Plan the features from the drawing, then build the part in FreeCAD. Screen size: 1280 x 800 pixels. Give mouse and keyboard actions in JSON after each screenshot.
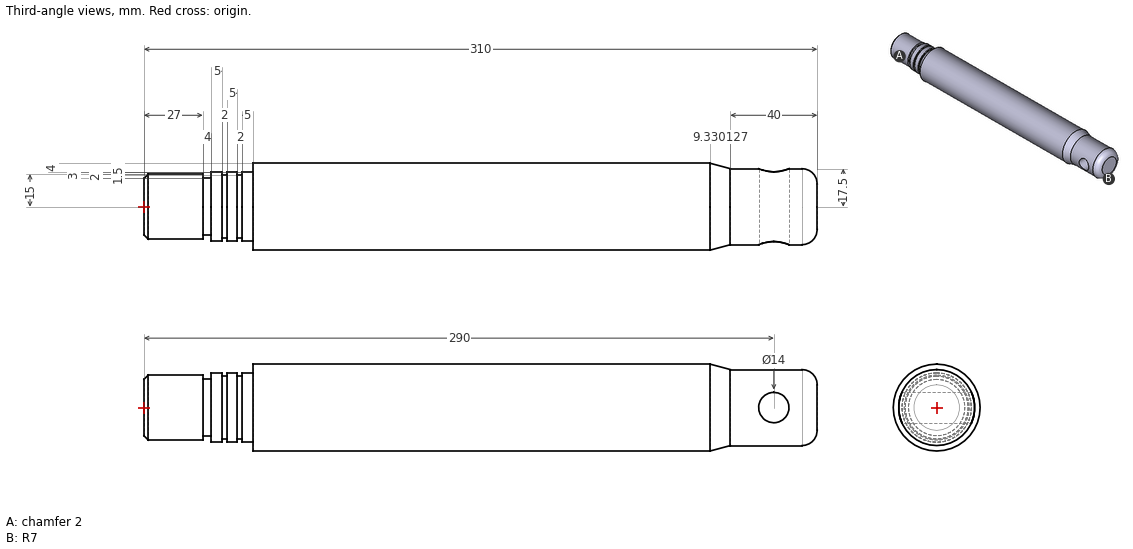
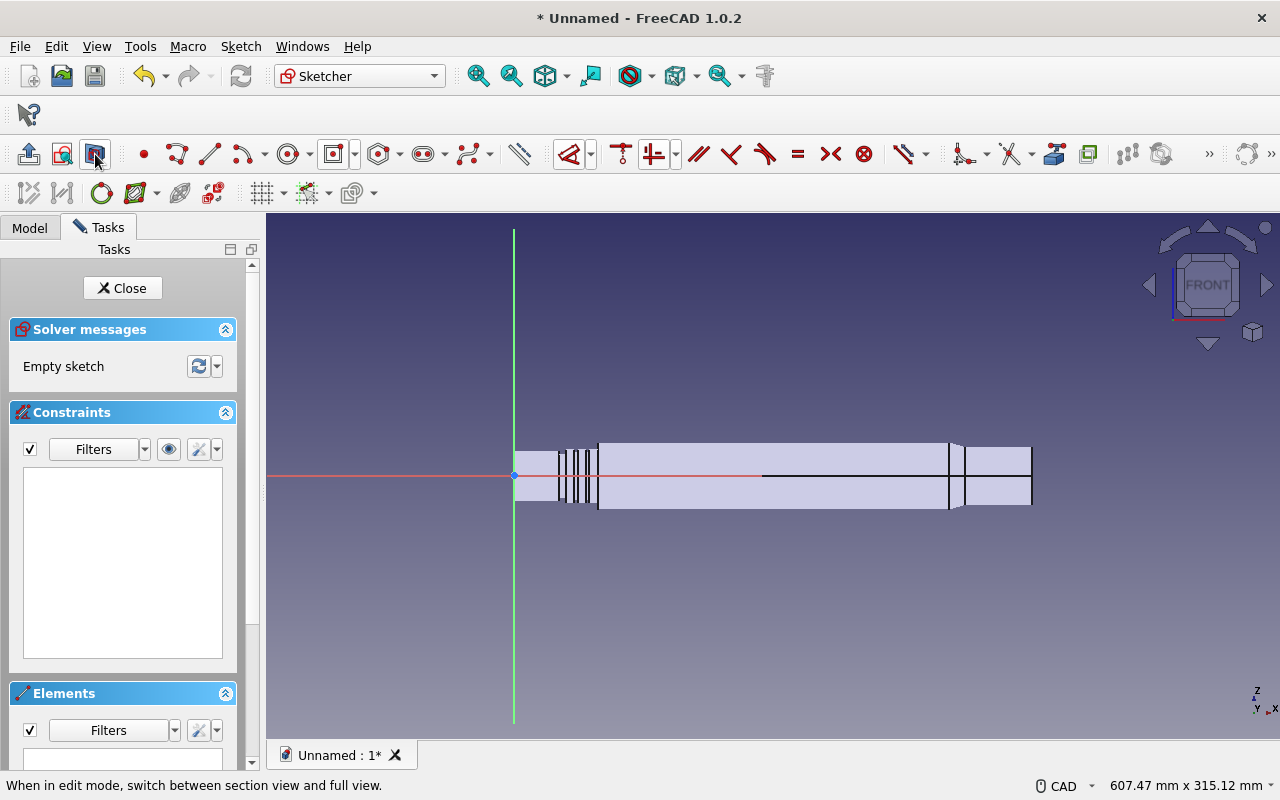
{"action": "scroll", "coordinate": [1022, 476], "scroll_direction": "up", "scroll_amount": 13}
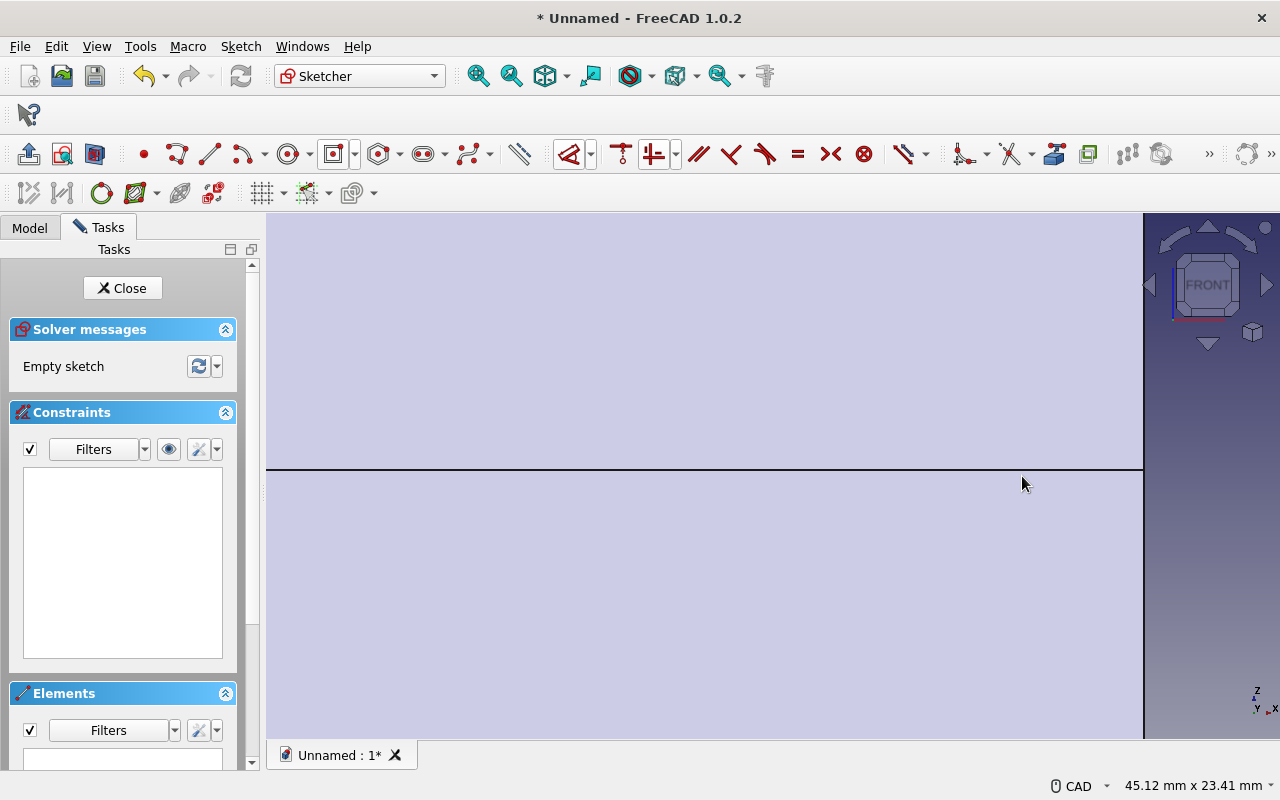
{"action": "left_click", "coordinate": [288, 154]}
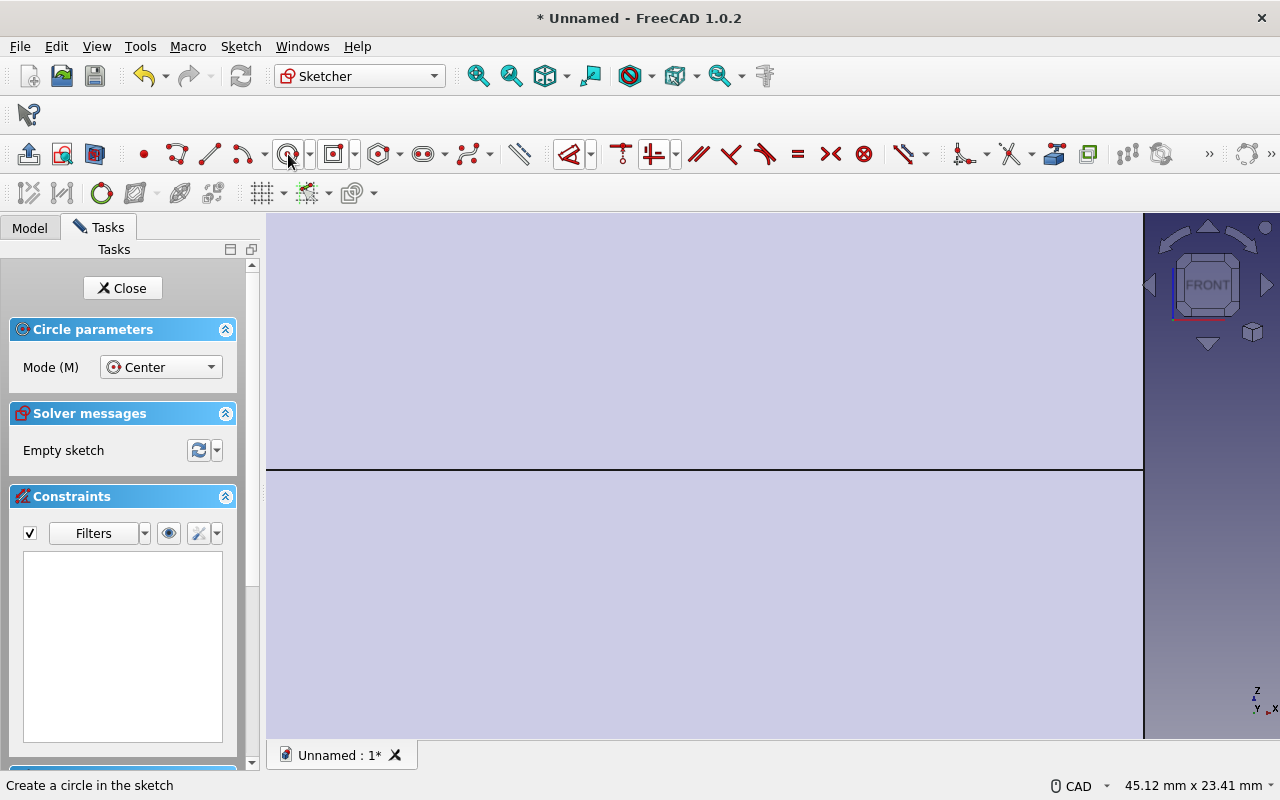
{"action": "left_click", "coordinate": [694, 470]}
{"action": "left_click", "coordinate": [805, 359]}
{"action": "key", "text": "Escape"}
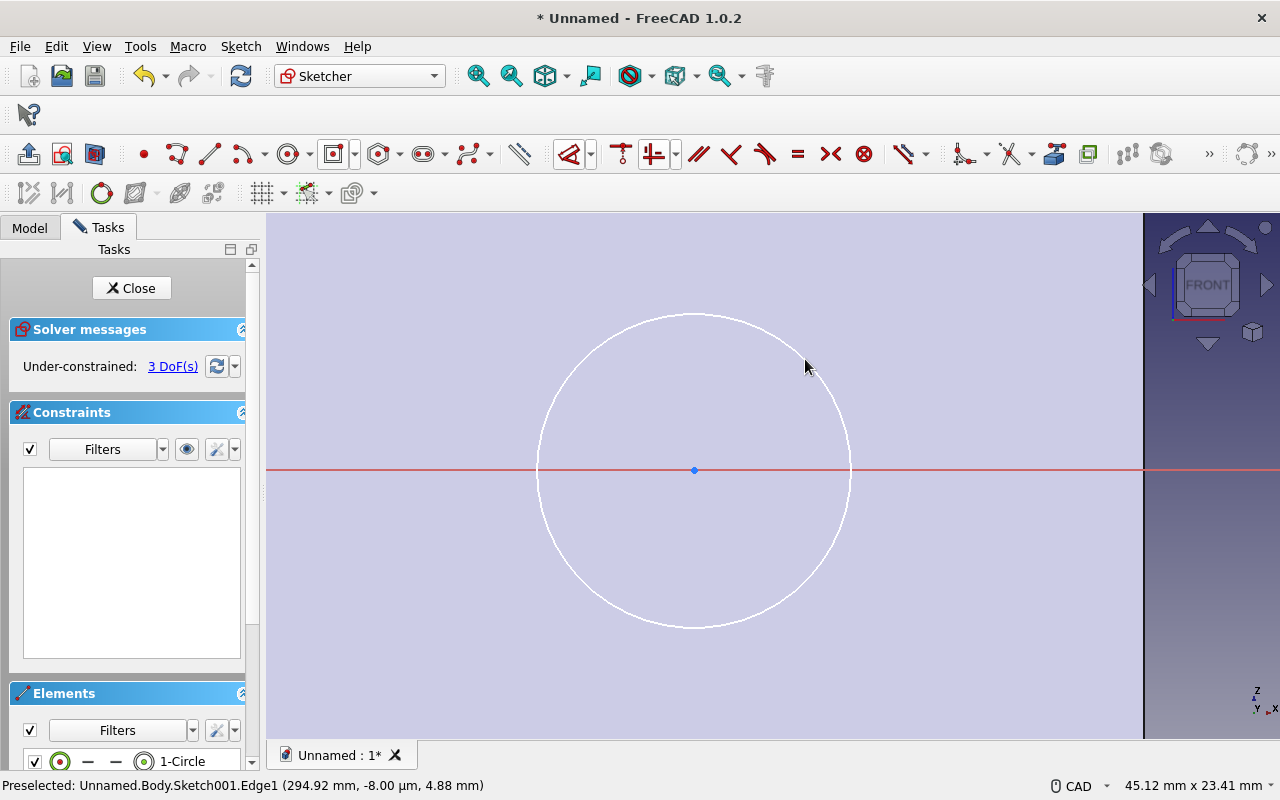
{"action": "left_click", "coordinate": [694, 471]}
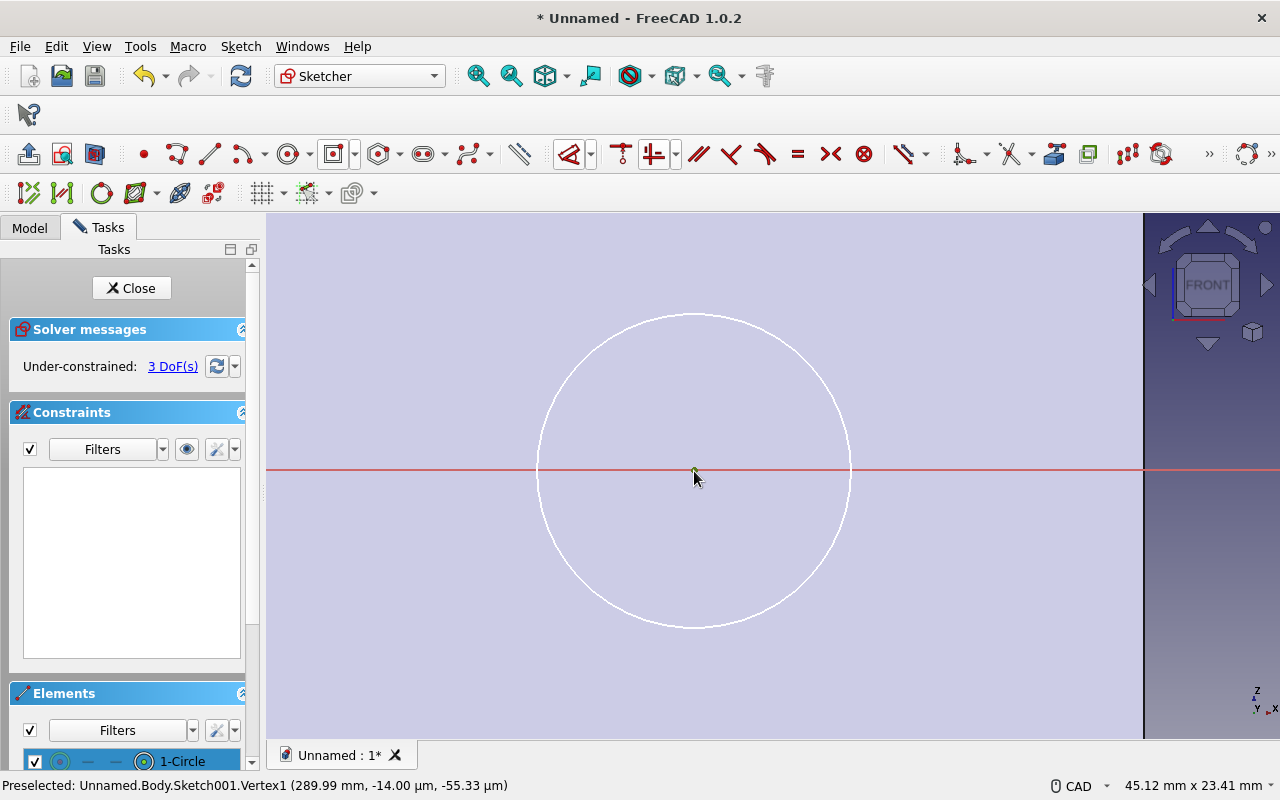
{"action": "left_click", "coordinate": [353, 470]}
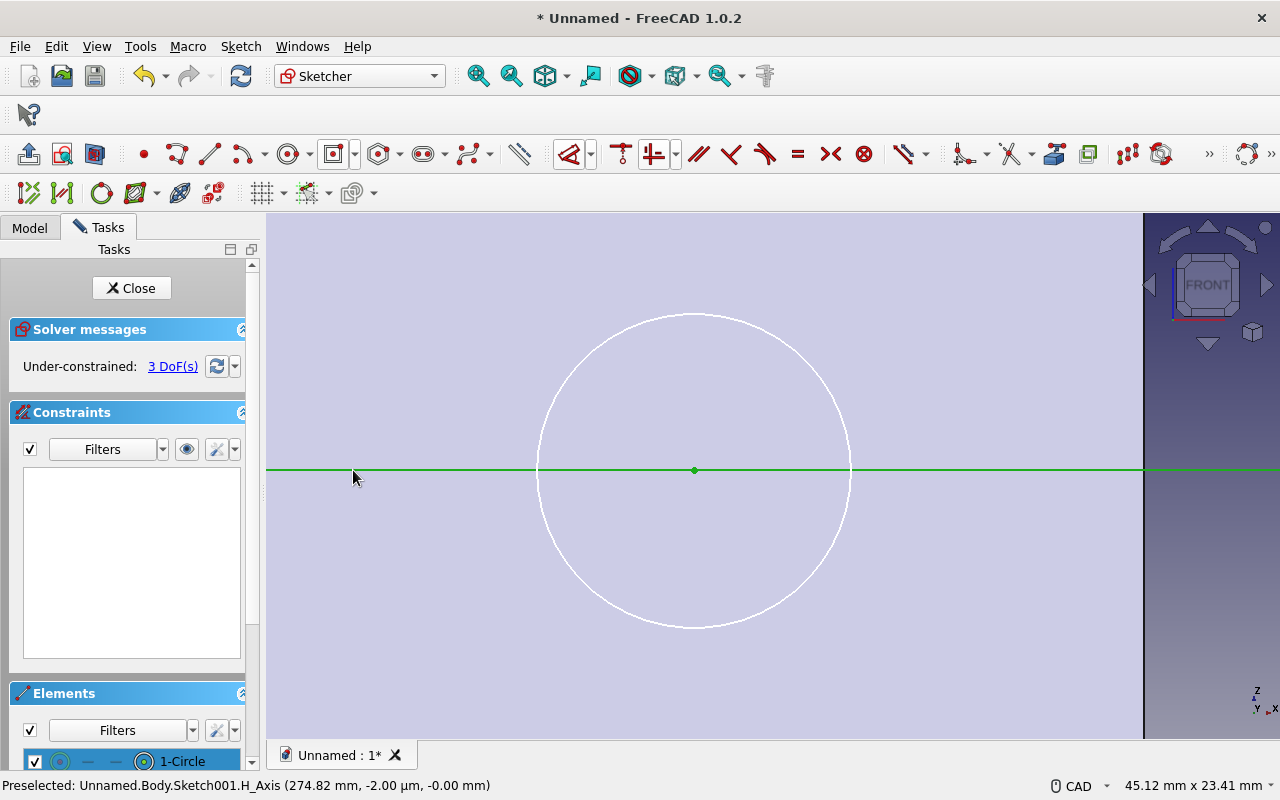
{"action": "left_click", "coordinate": [621, 154]}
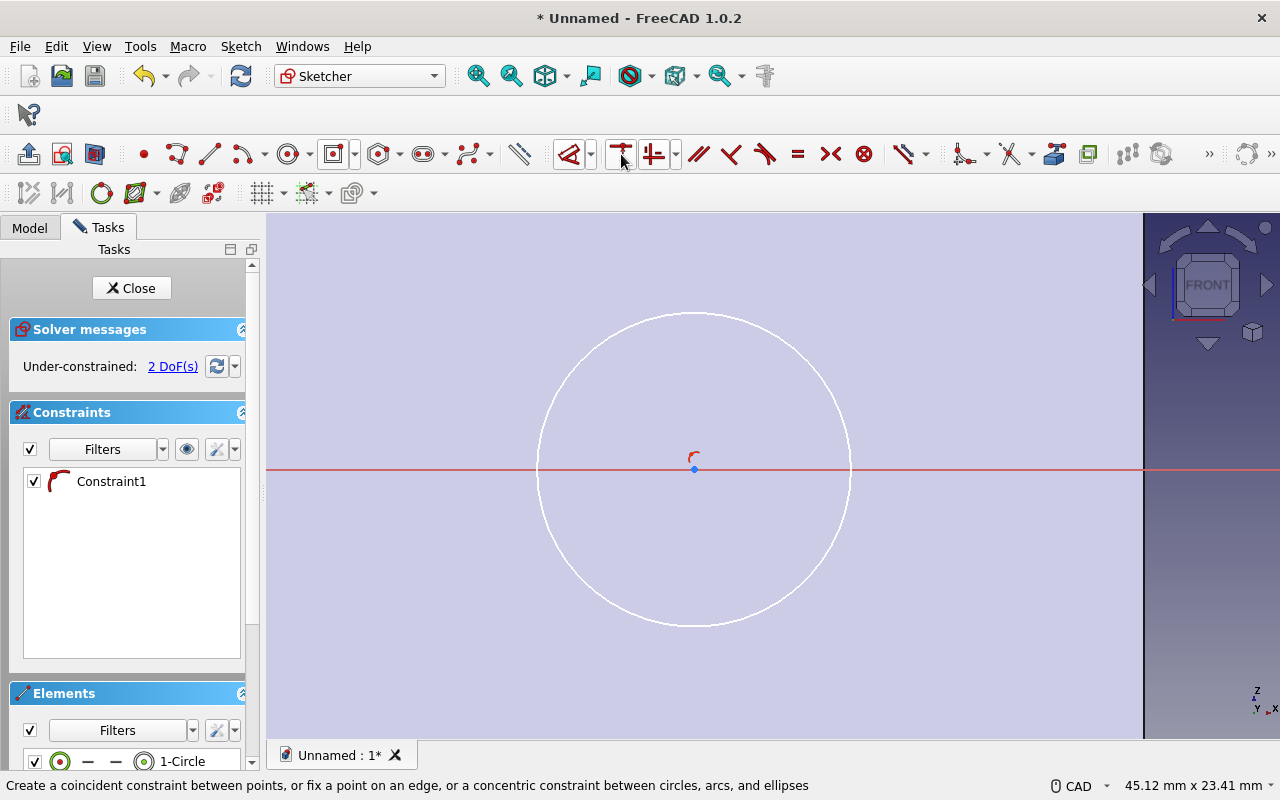
{"action": "left_click", "coordinate": [805, 358]}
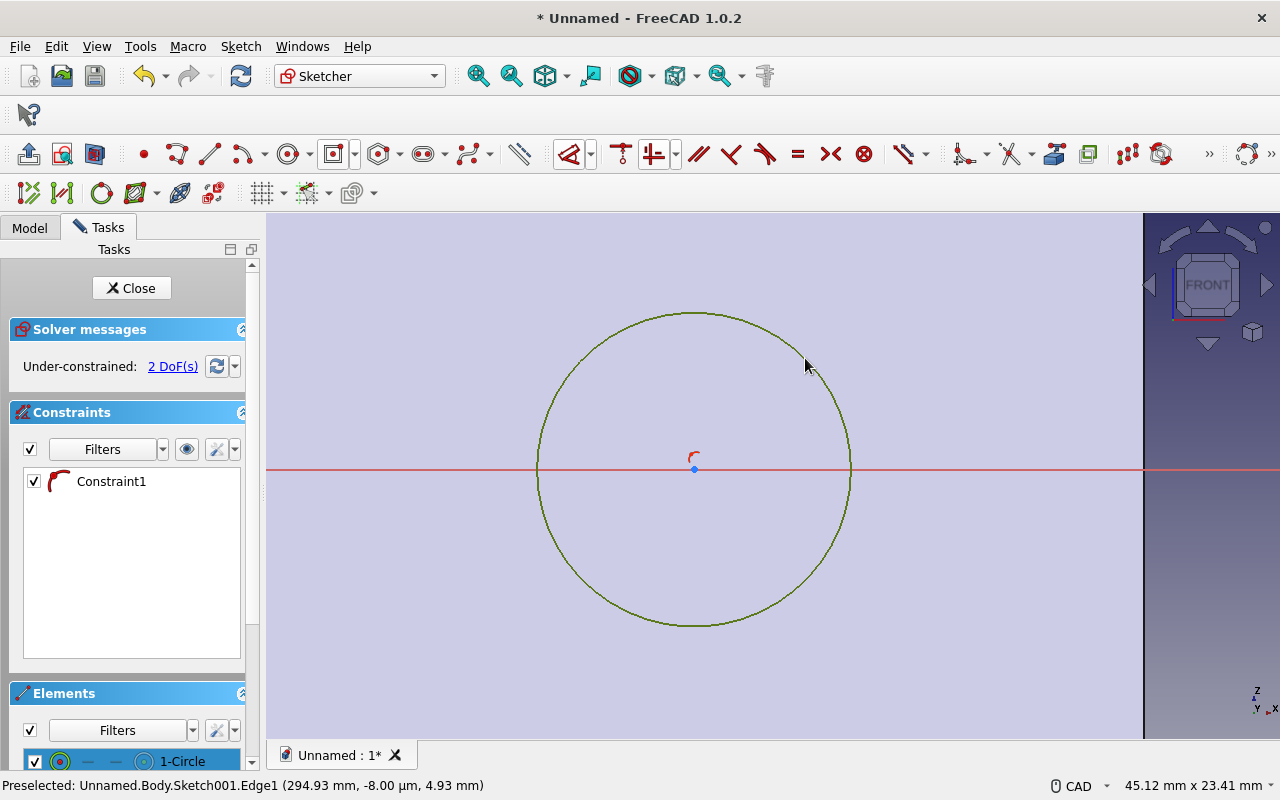
{"action": "left_click", "coordinate": [590, 154]}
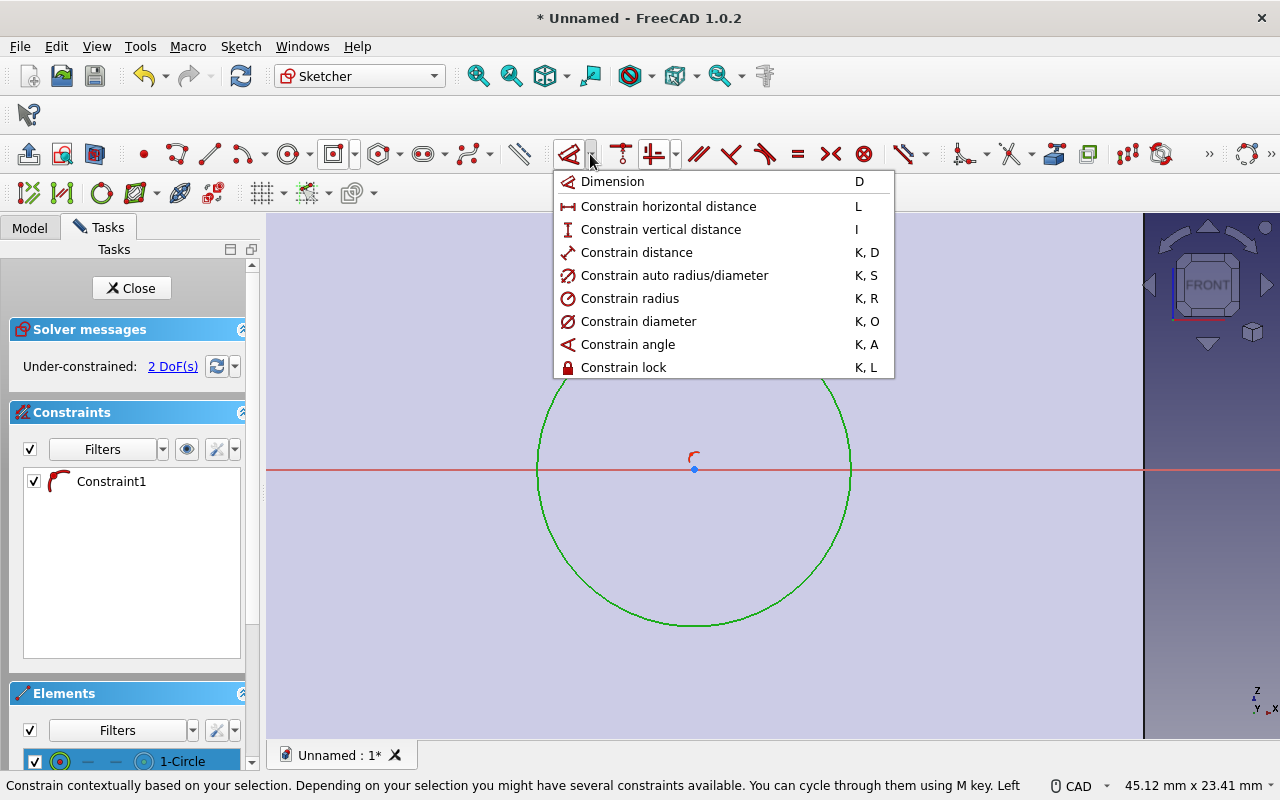
{"action": "left_click", "coordinate": [724, 322]}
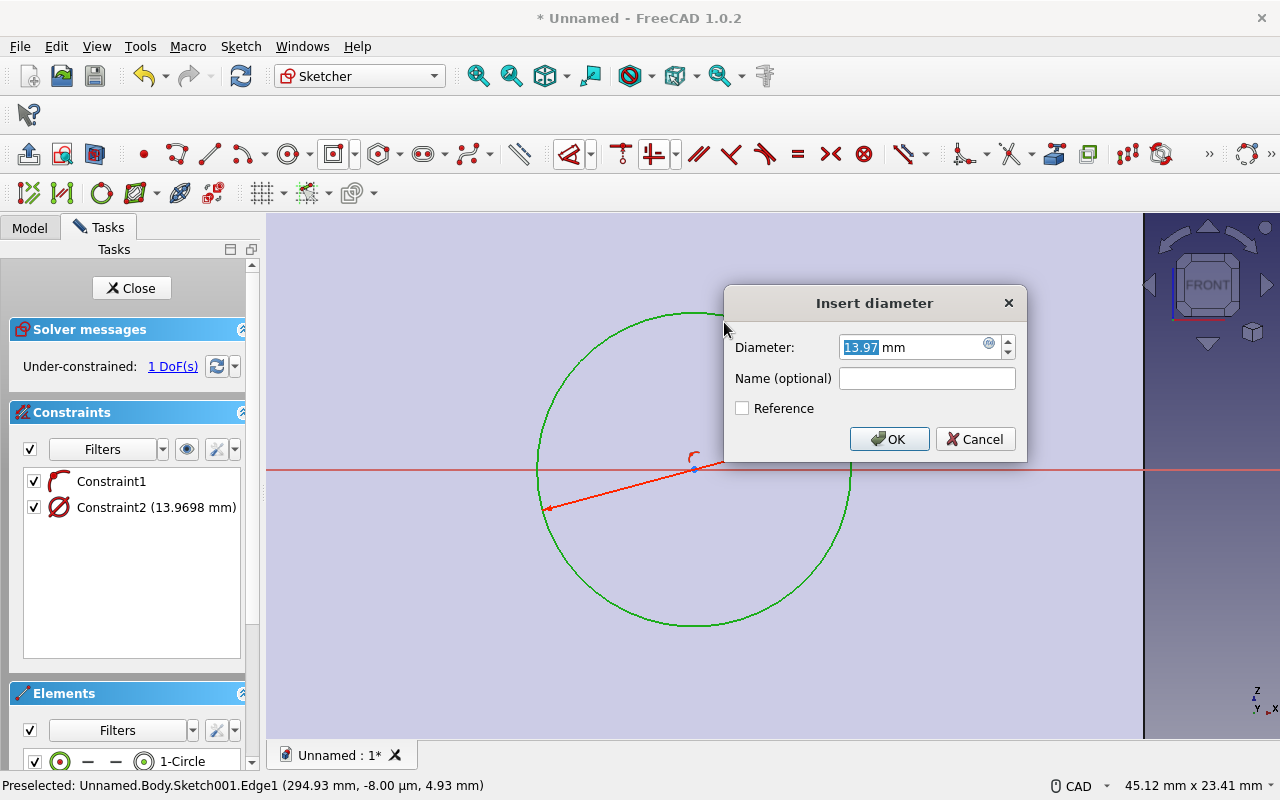
{"action": "type", "text": "14"}
{"action": "key", "text": "Return"}